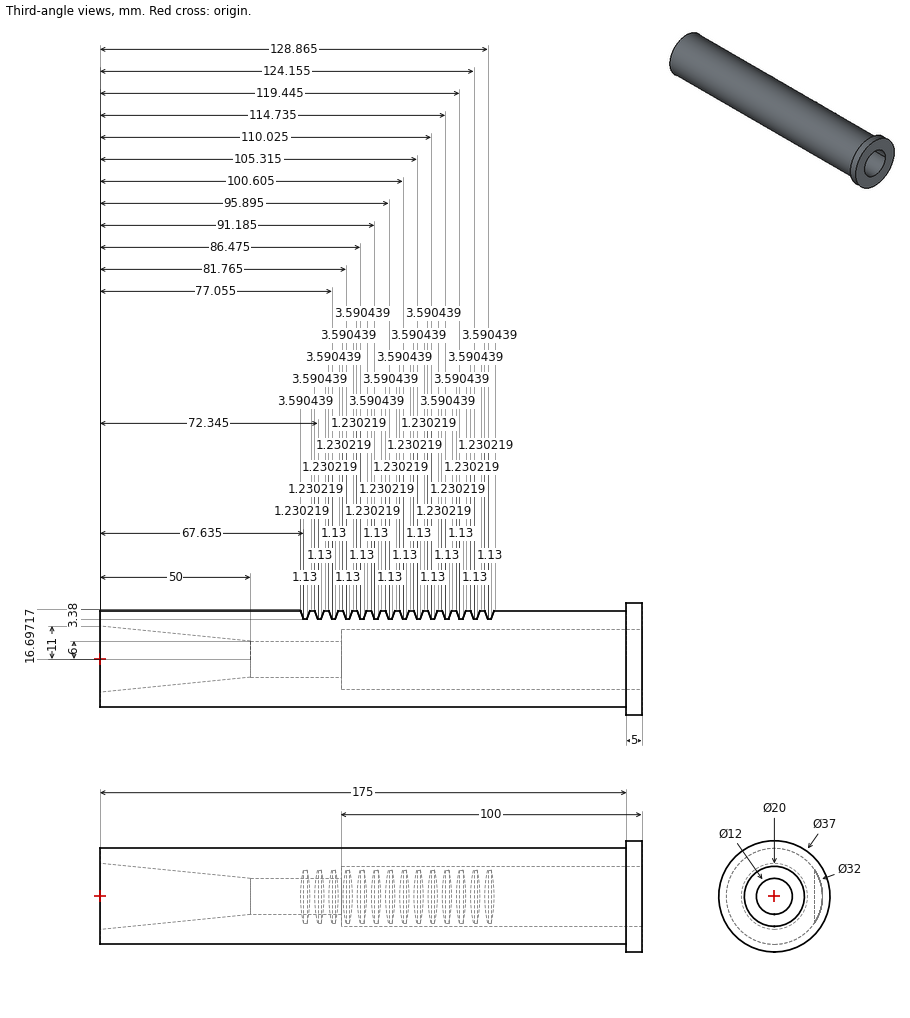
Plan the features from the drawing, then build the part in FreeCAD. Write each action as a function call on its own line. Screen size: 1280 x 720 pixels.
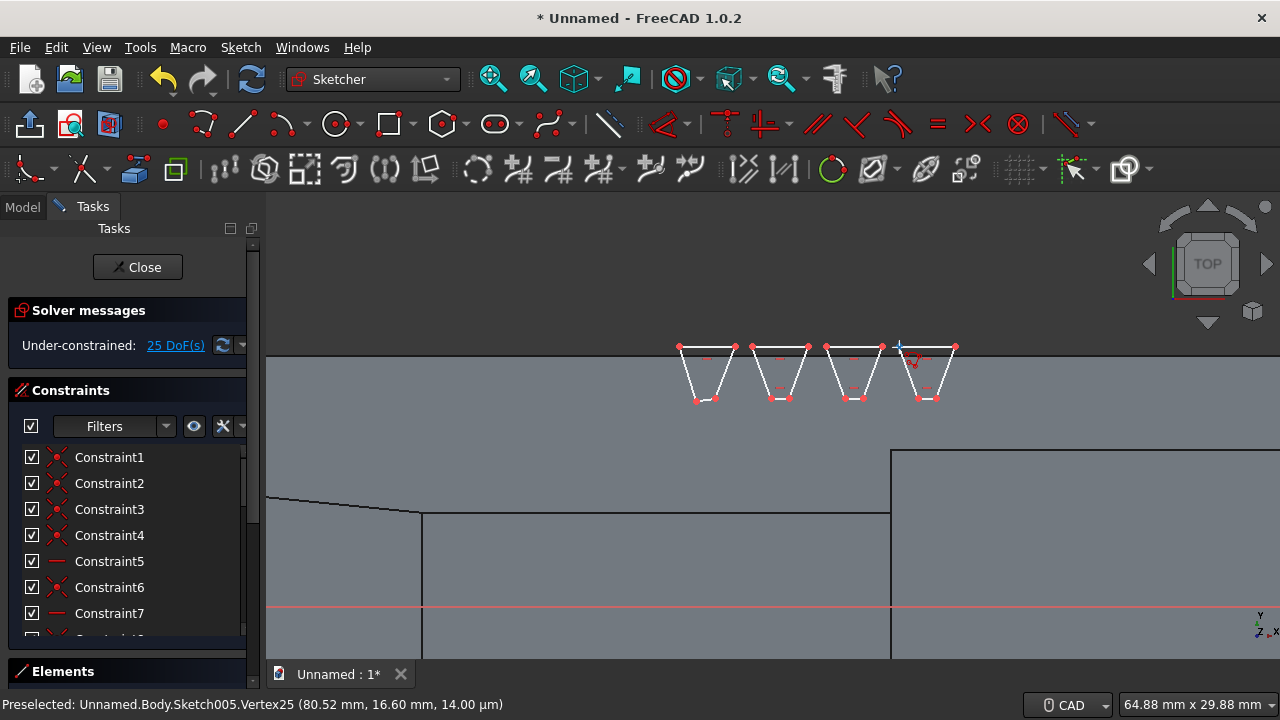
click(973, 346)
click(992, 398)
click(1010, 398)
click(1029, 346)
click(973, 347)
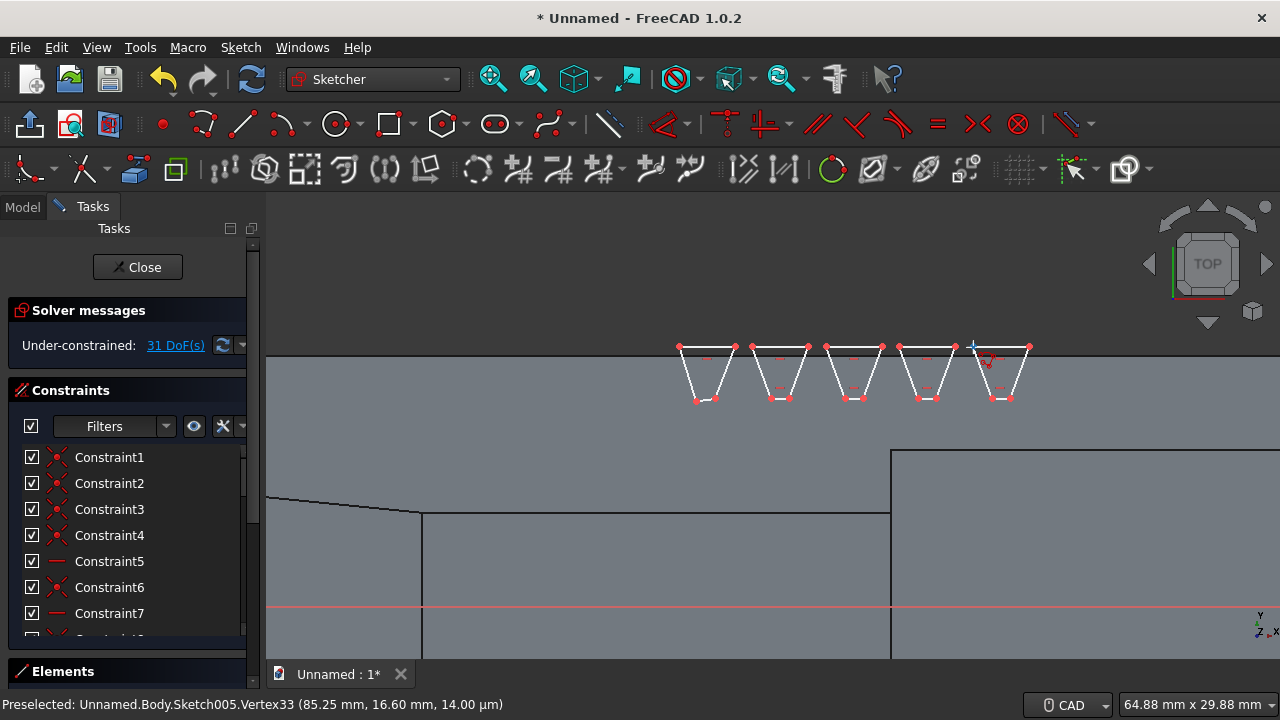
click(1046, 346)
click(1066, 398)
click(1083, 398)
click(1103, 346)
click(1046, 347)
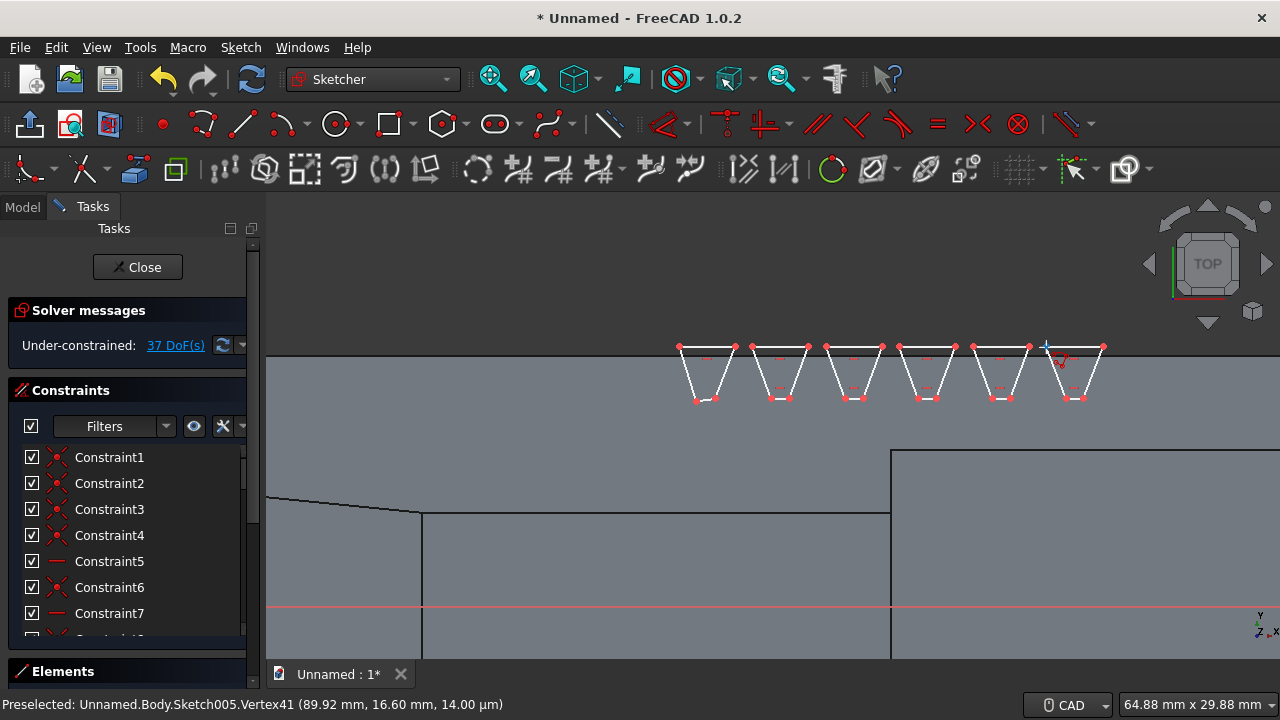
scroll(721, 404, down, 6)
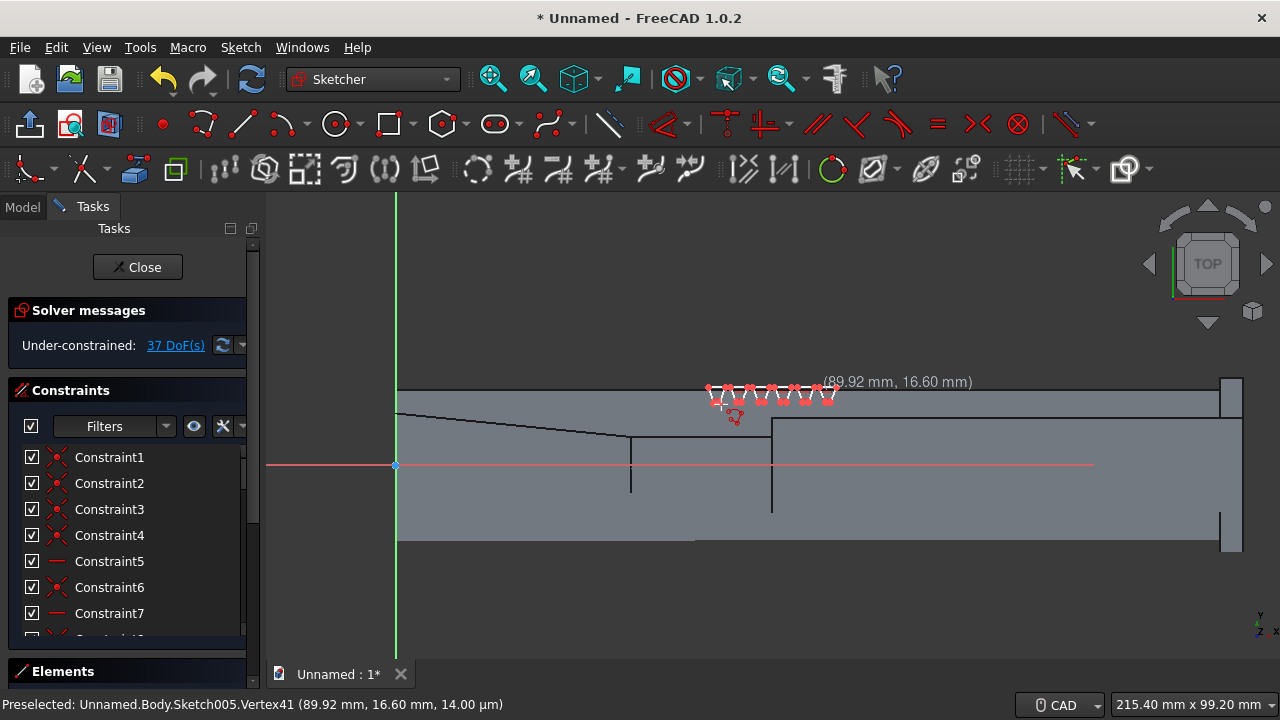
scroll(842, 387, up, 6)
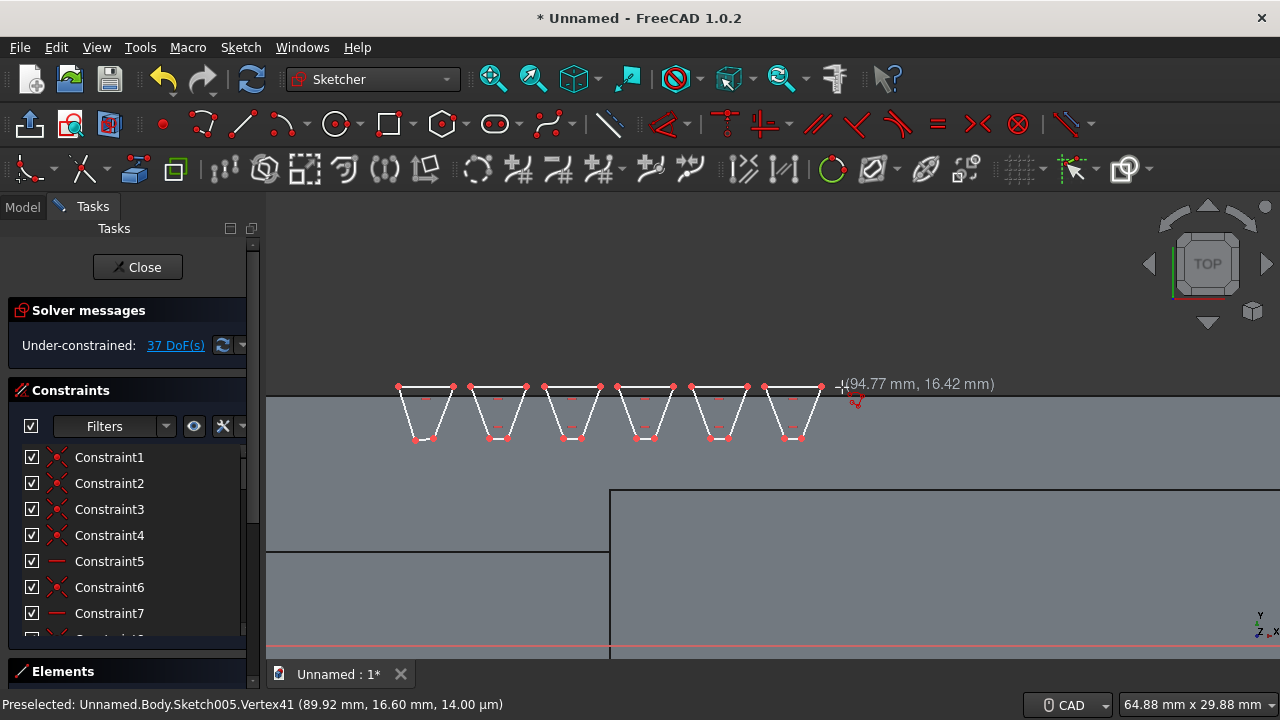
click(839, 385)
click(858, 438)
click(876, 438)
click(895, 385)
click(839, 386)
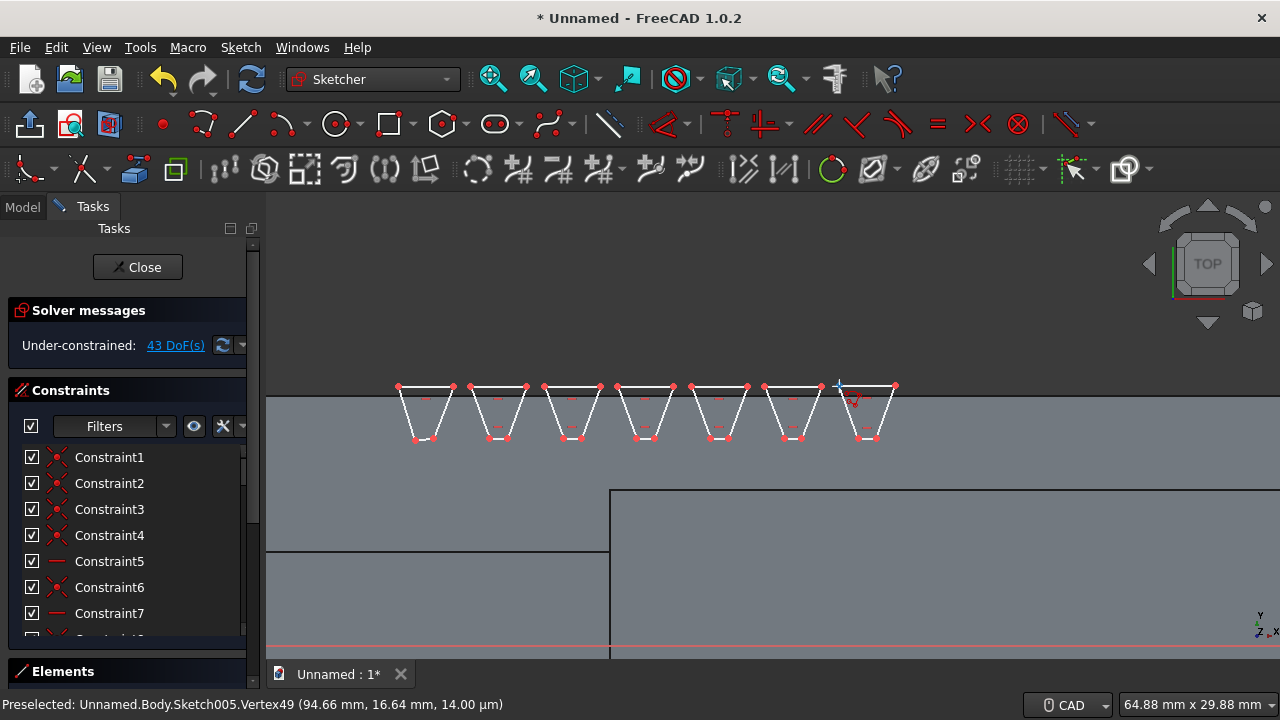
click(913, 385)
click(932, 438)
click(950, 438)
click(969, 385)
click(913, 386)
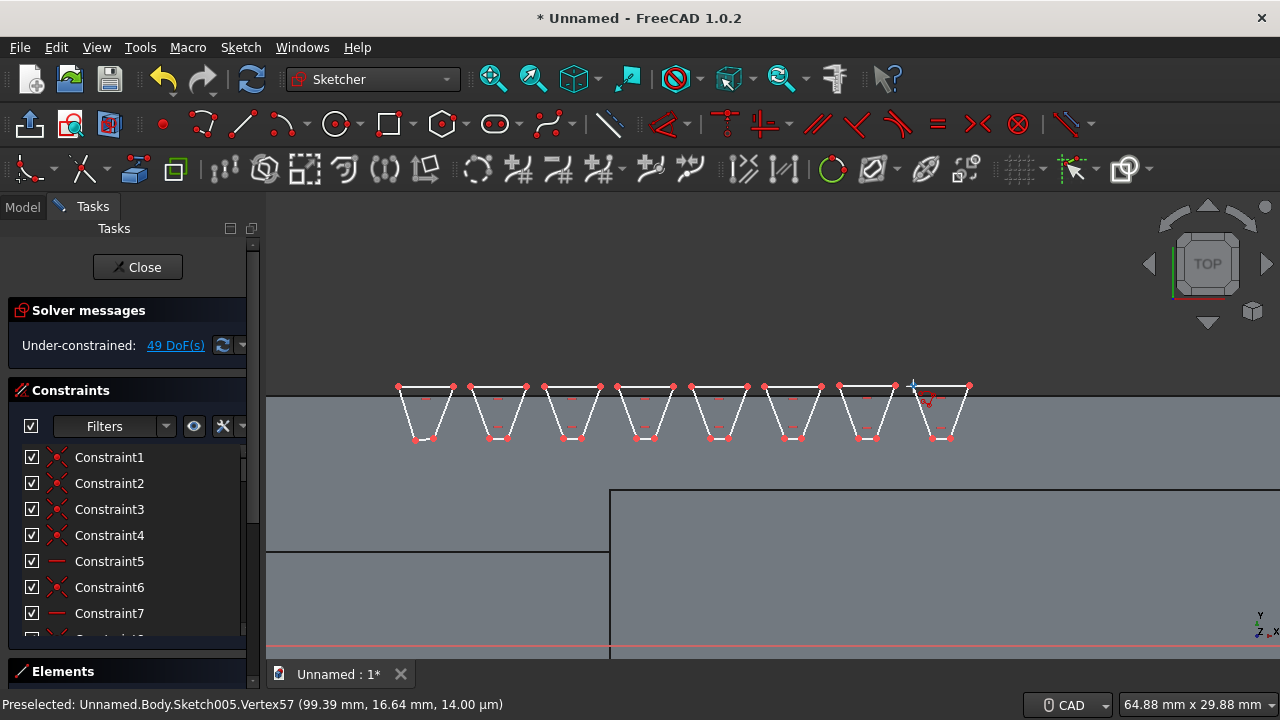
click(986, 385)
click(1006, 438)
click(1023, 438)
click(1042, 385)
click(986, 386)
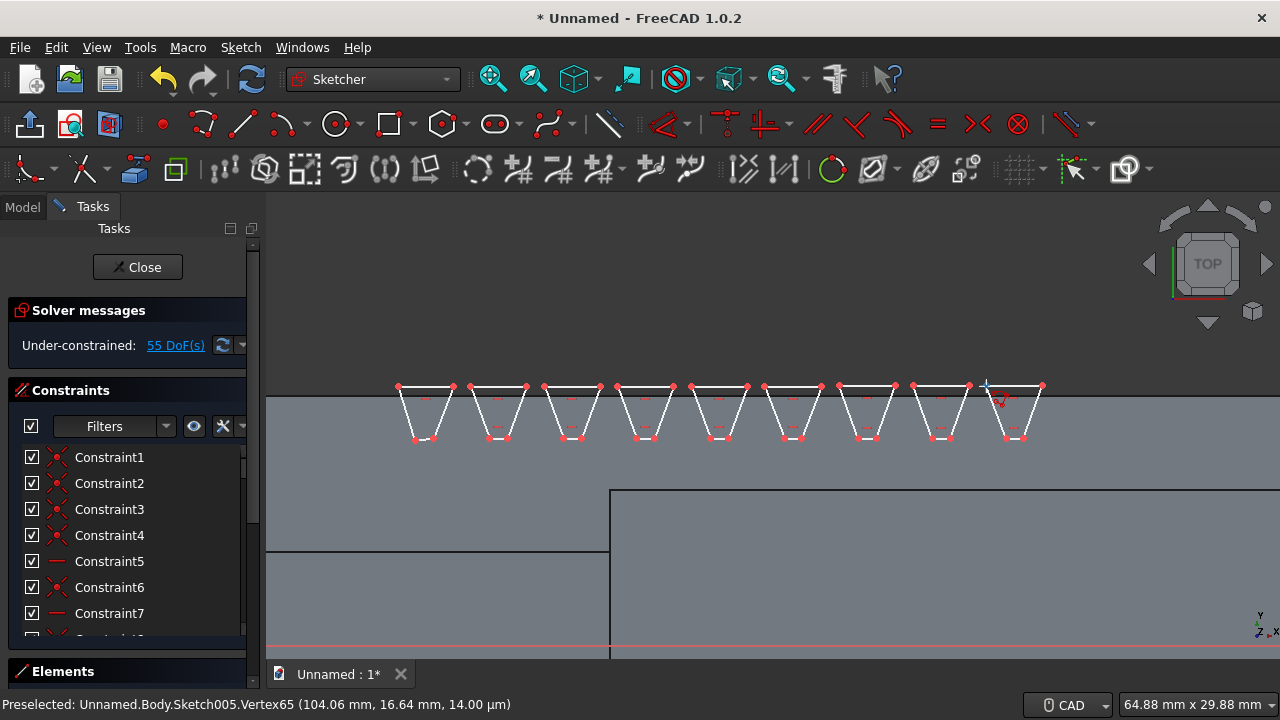
click(1060, 385)
click(1079, 438)
click(1097, 438)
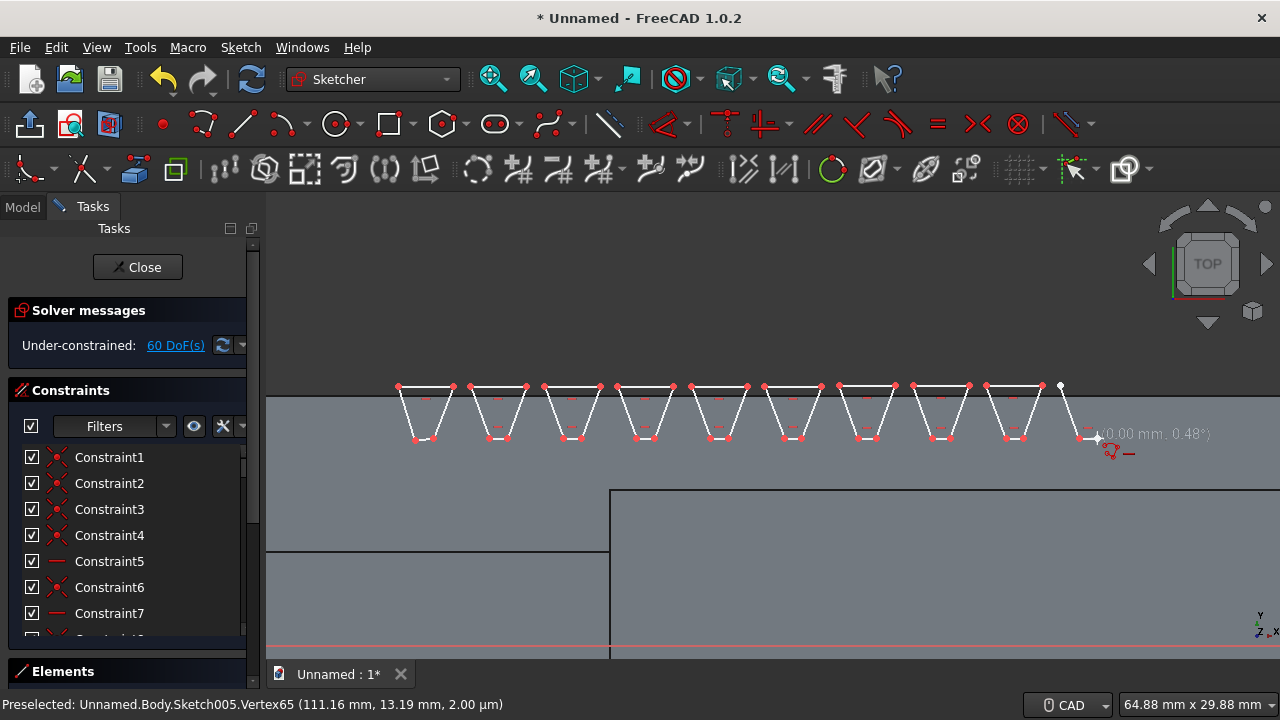
scroll(842, 387, down, 6)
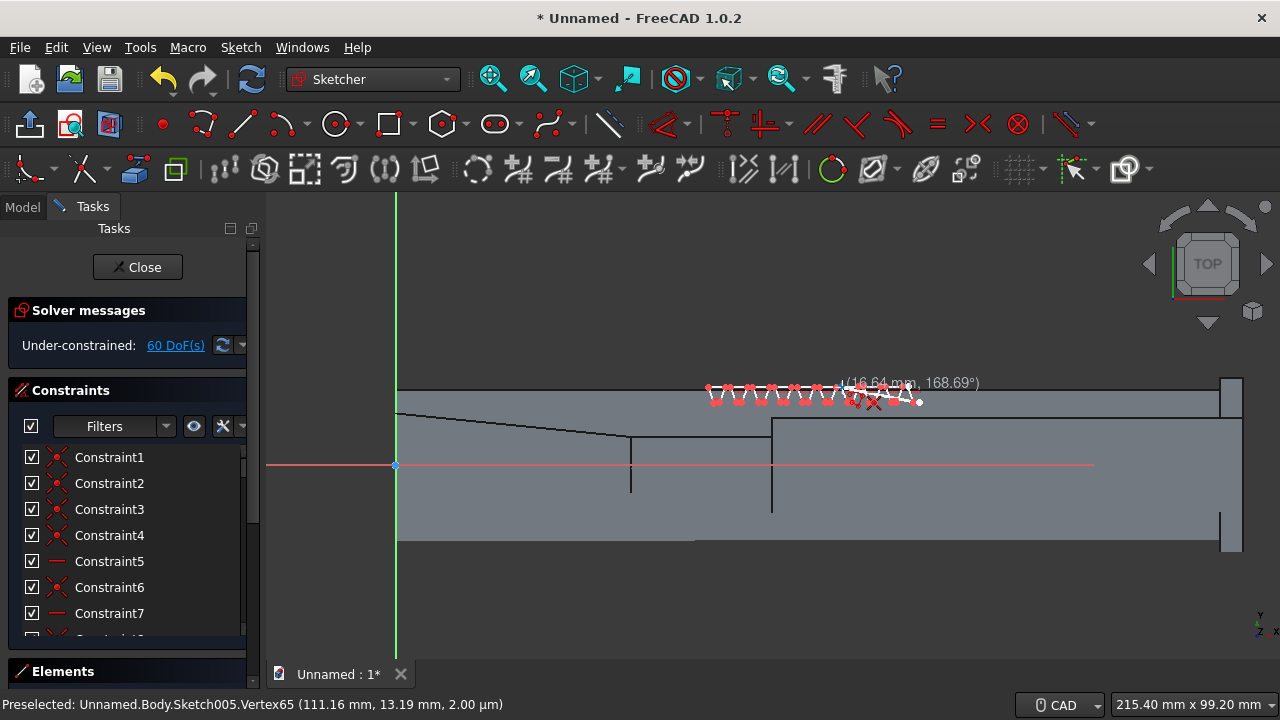
click(925, 387)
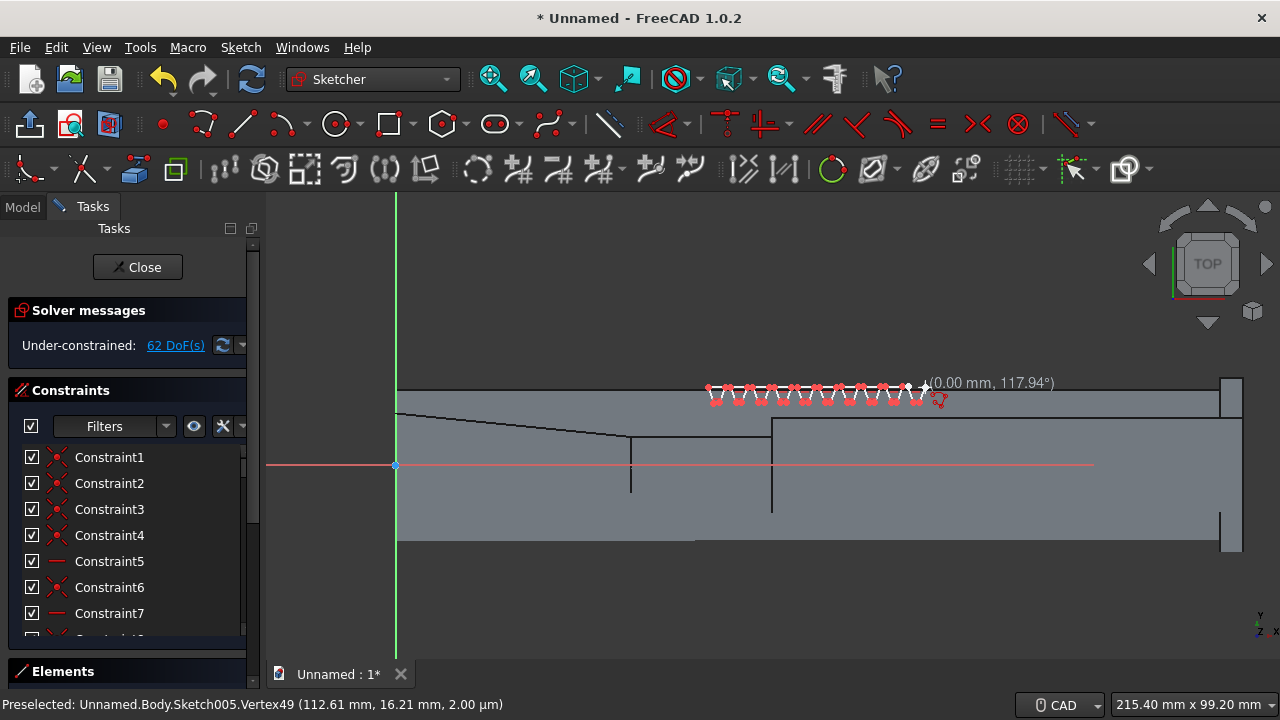
scroll(908, 387, up, 6)